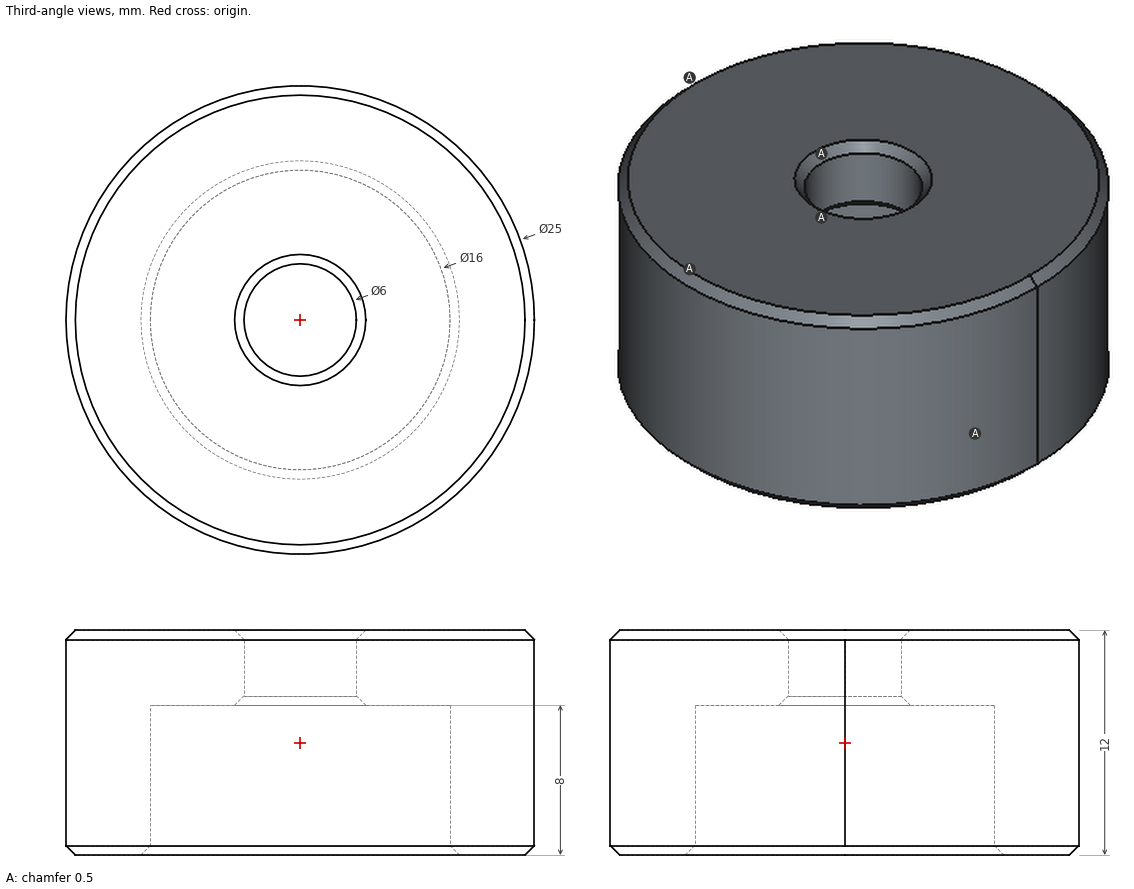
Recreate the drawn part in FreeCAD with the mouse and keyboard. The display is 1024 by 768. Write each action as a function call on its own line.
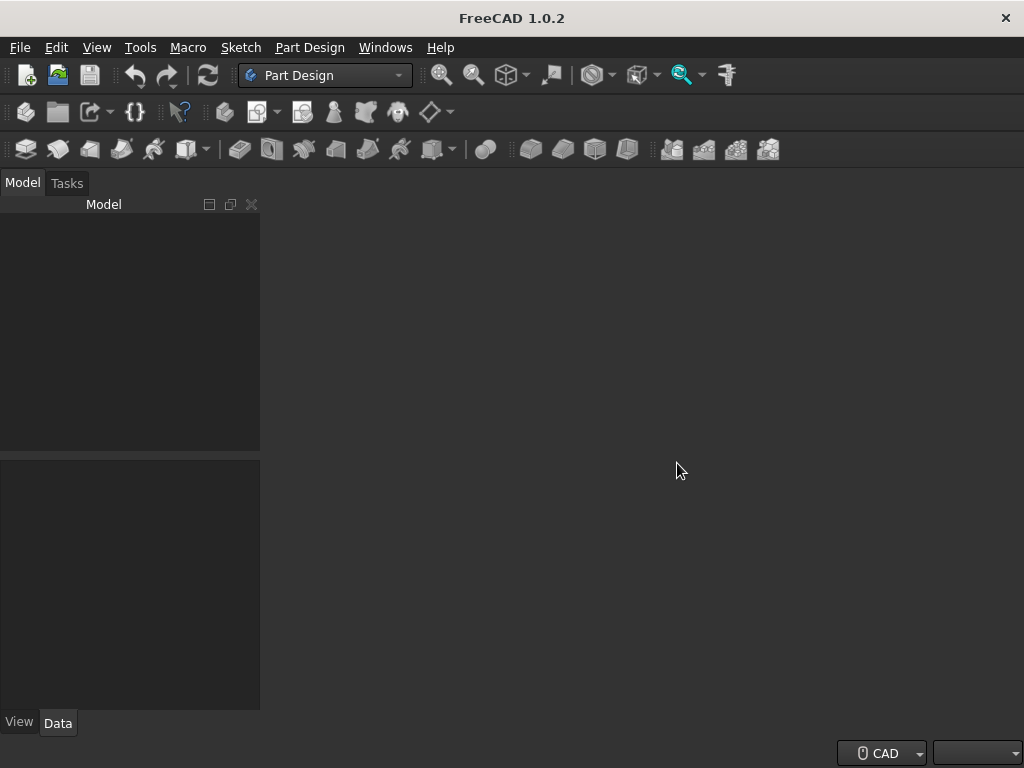
key(ctrl+n)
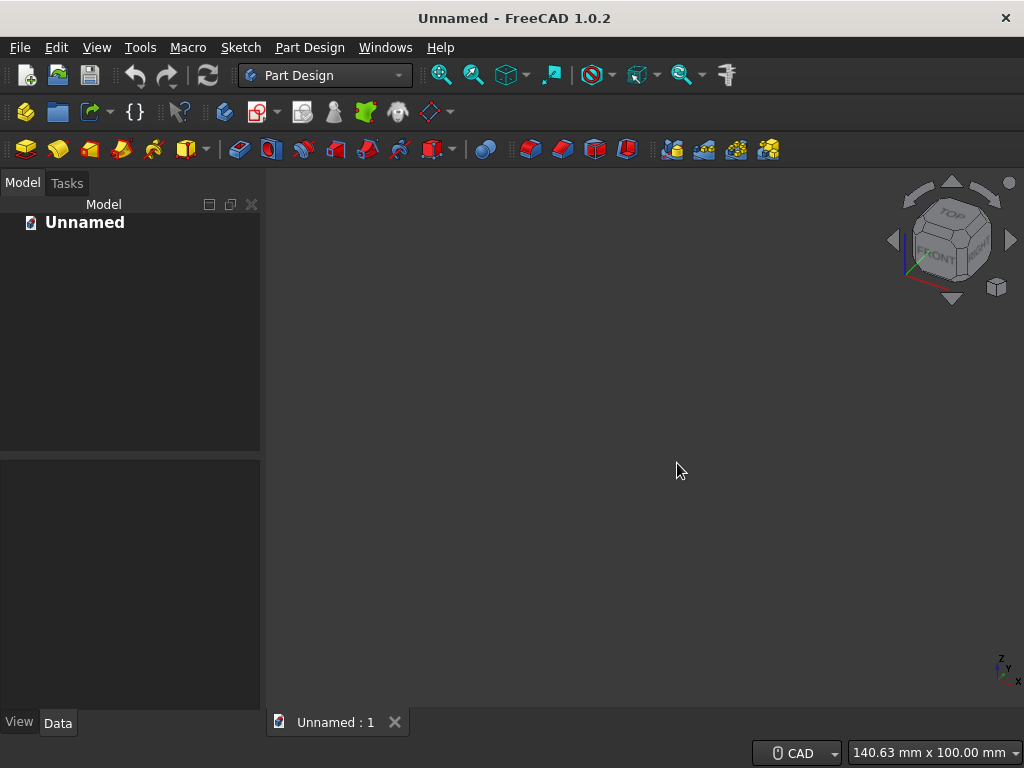
click(258, 112)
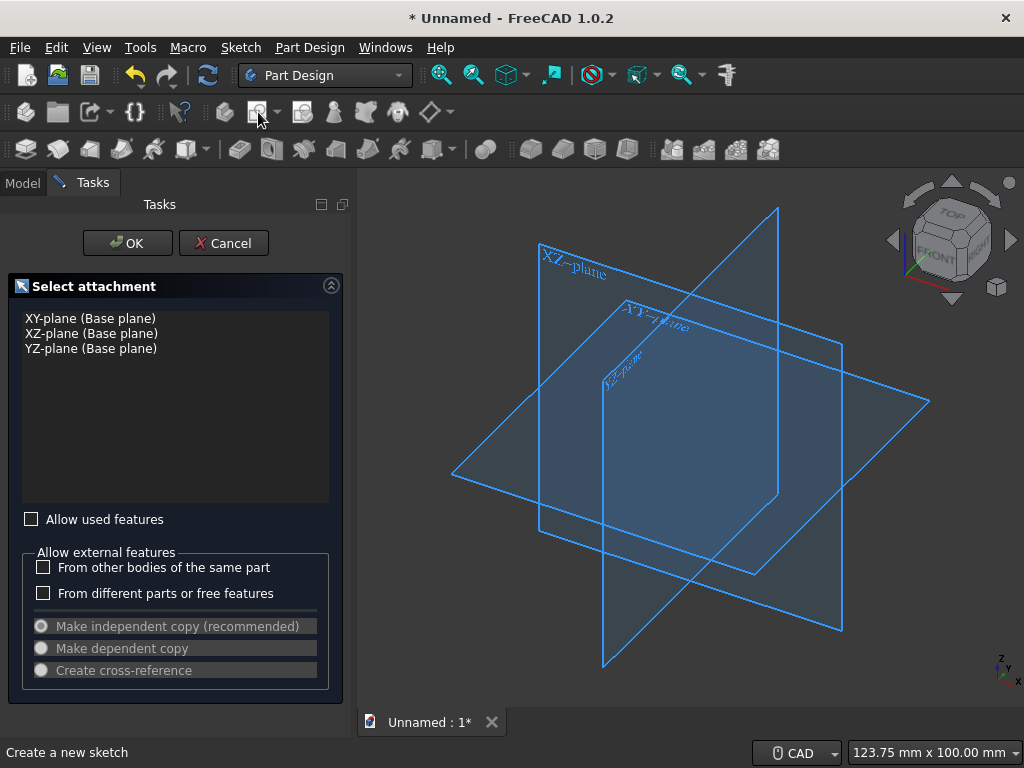
click(82, 318)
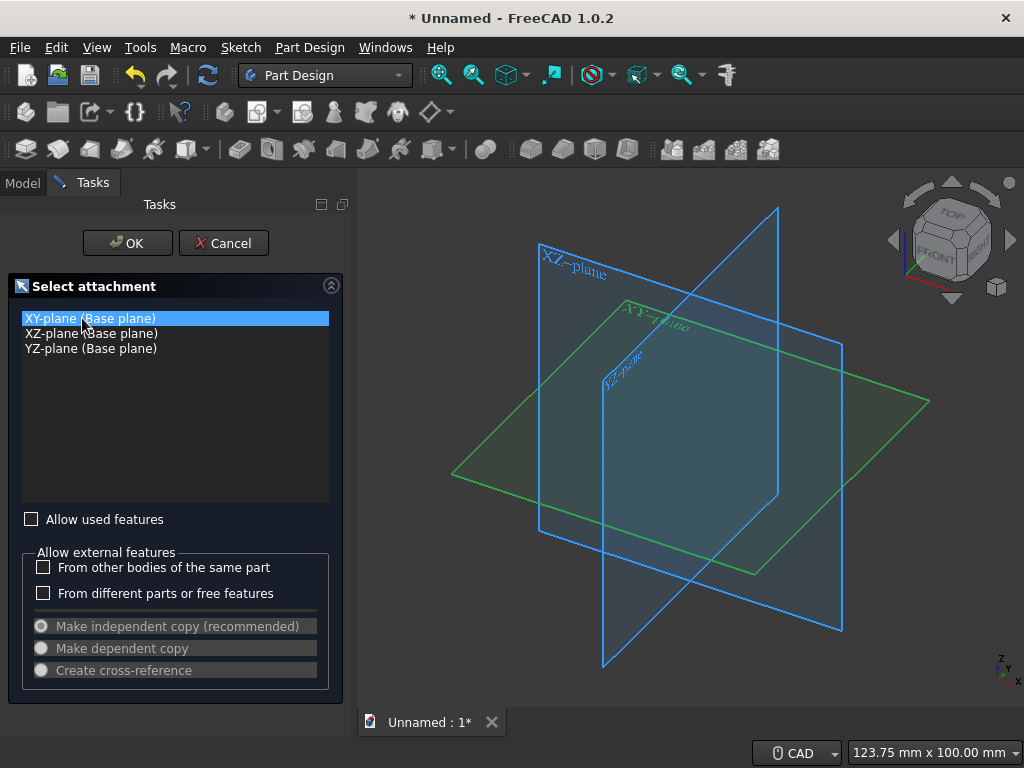
click(128, 243)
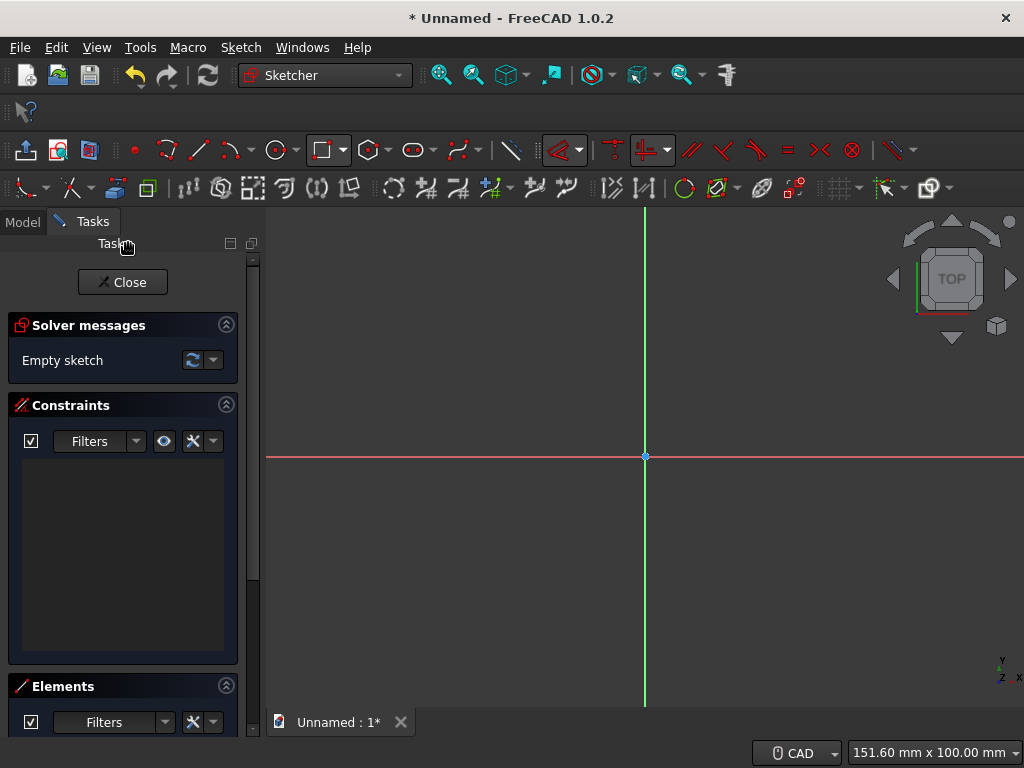
scroll(685, 457, up, 5)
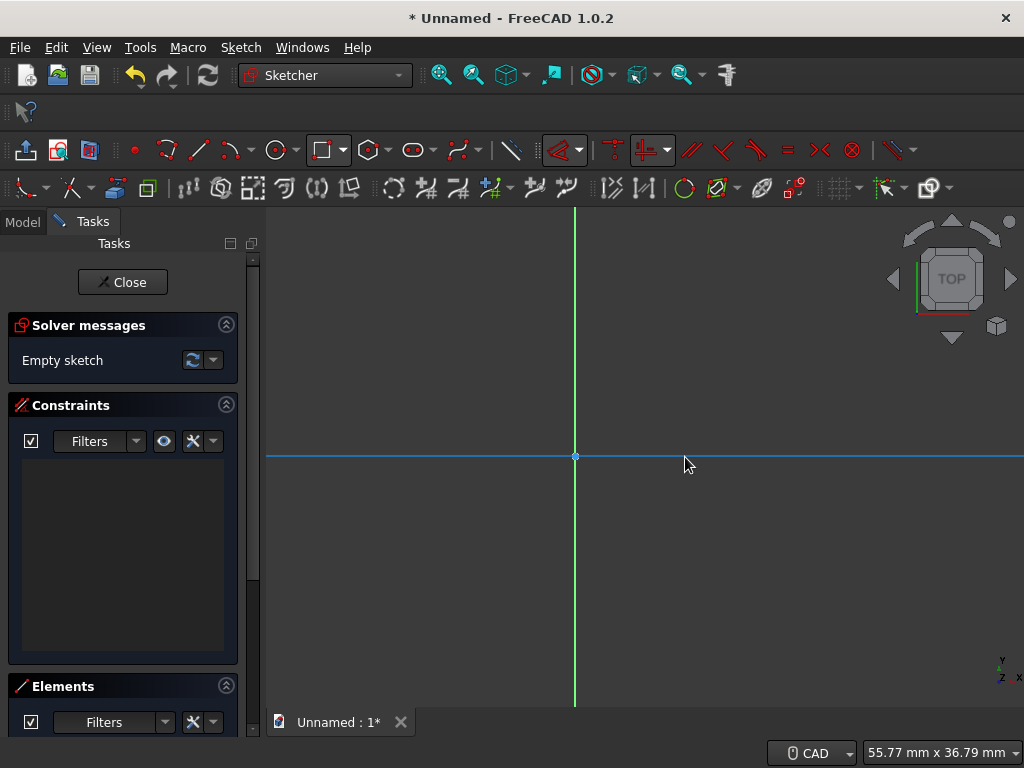
key(g)
key(c)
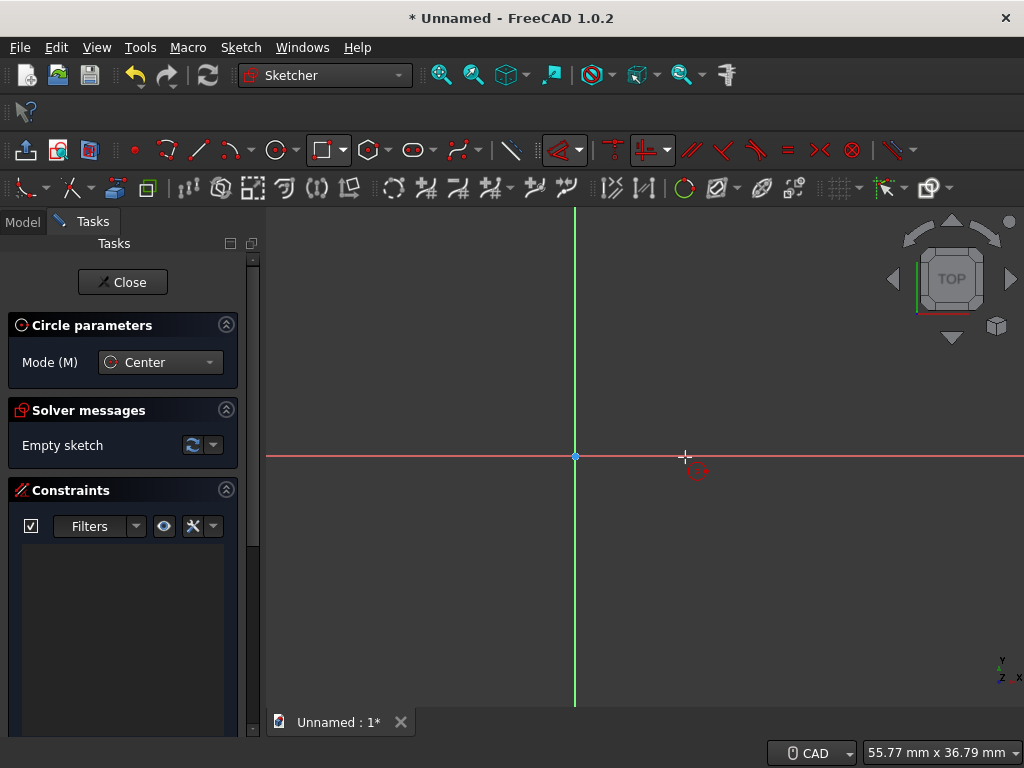
click(575, 456)
move(695, 336)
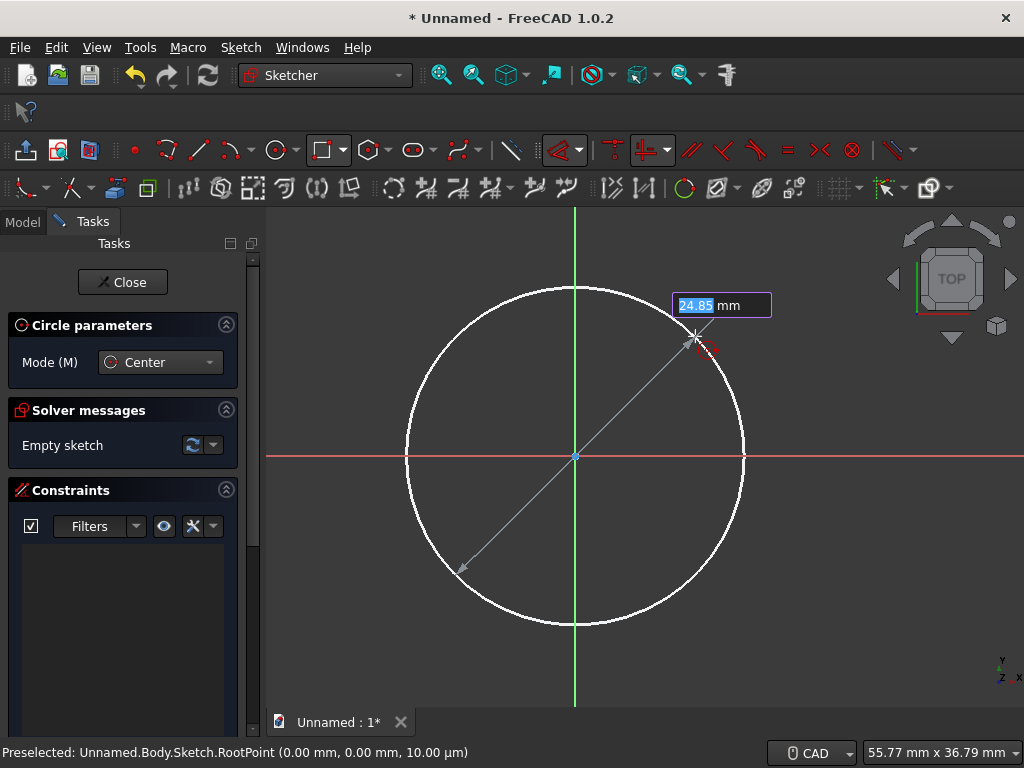
text(25)
key(Return)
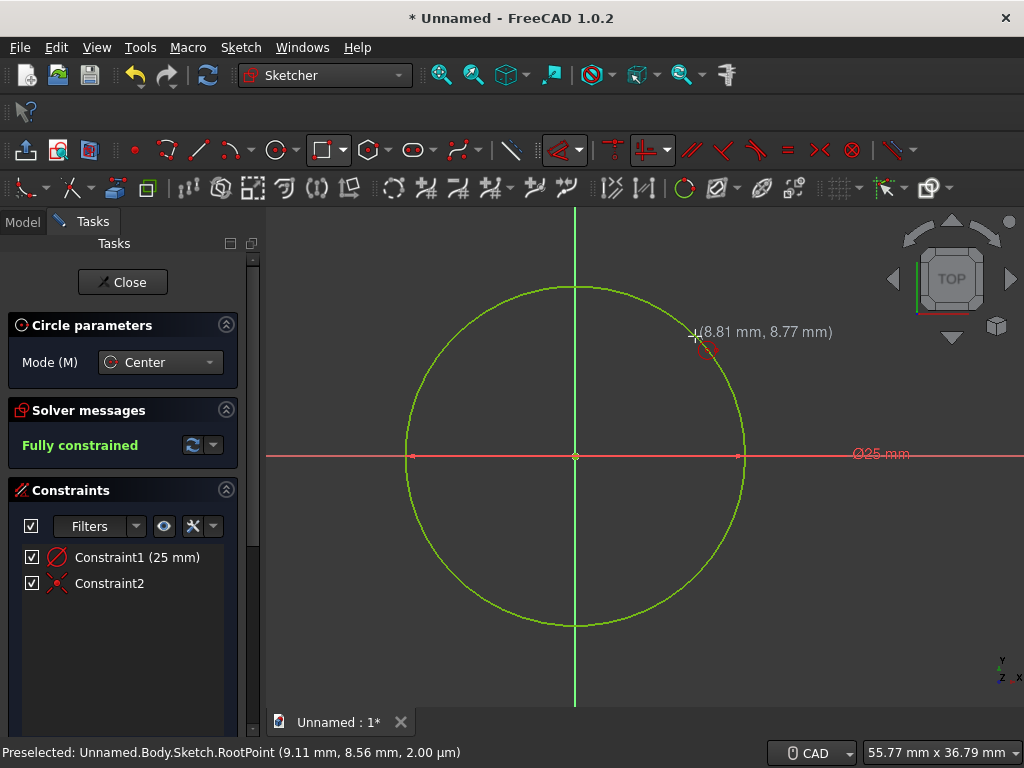
click(575, 456)
move(604, 427)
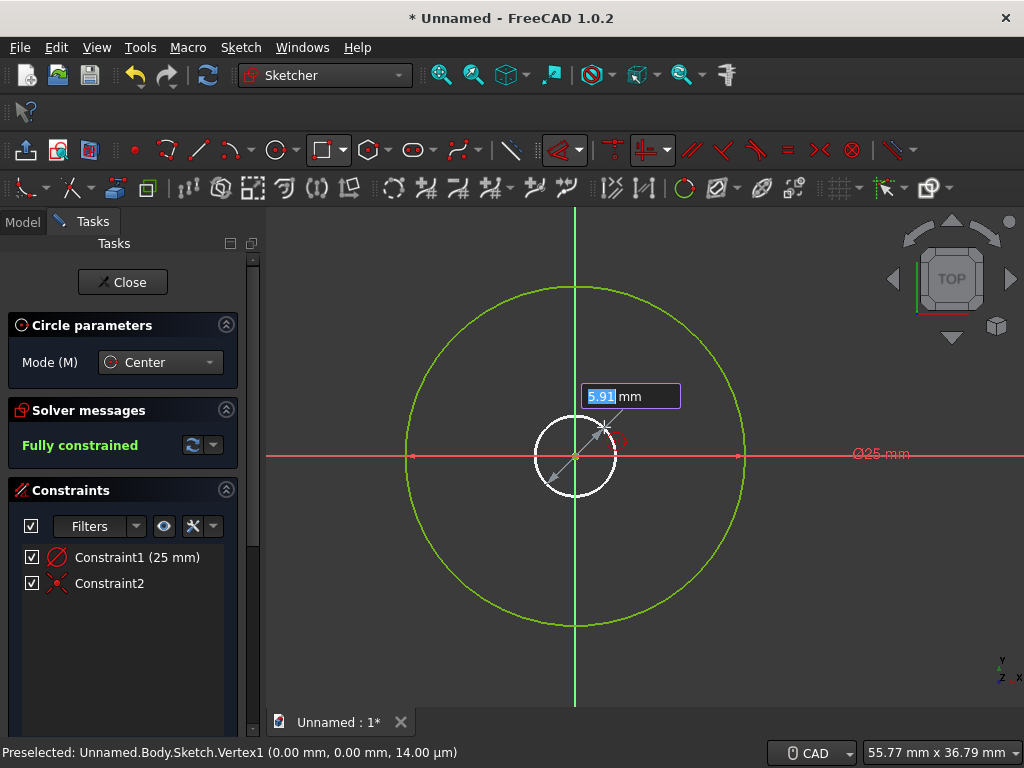
text(6)
key(Return)
key(Escape)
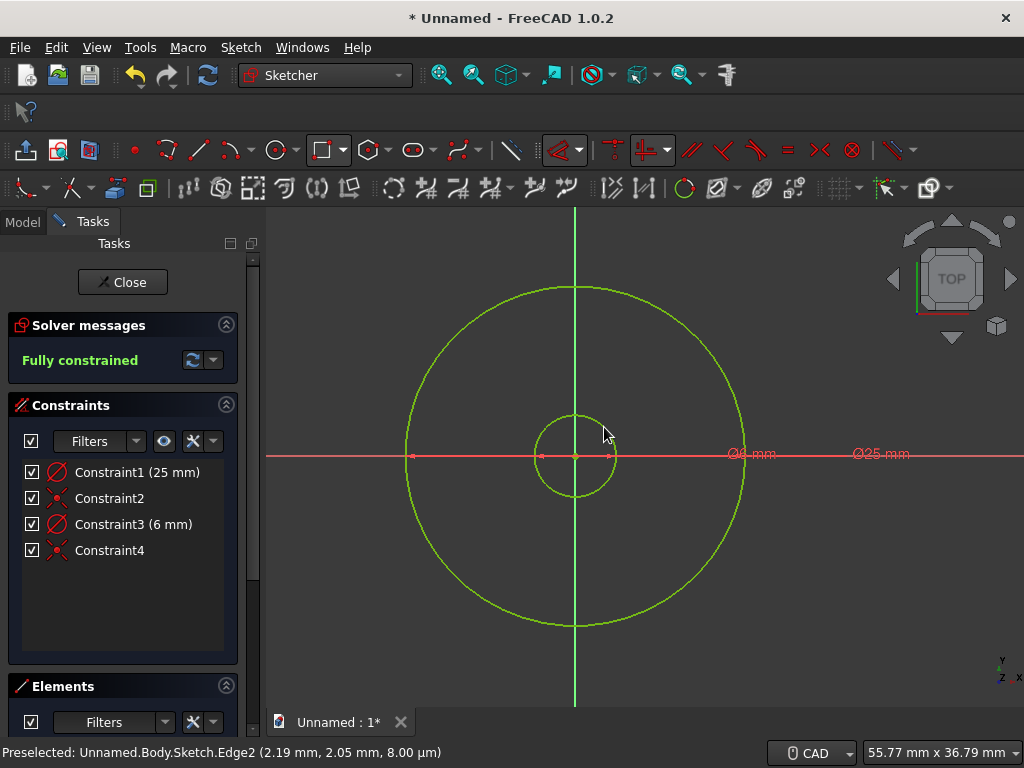
click(123, 282)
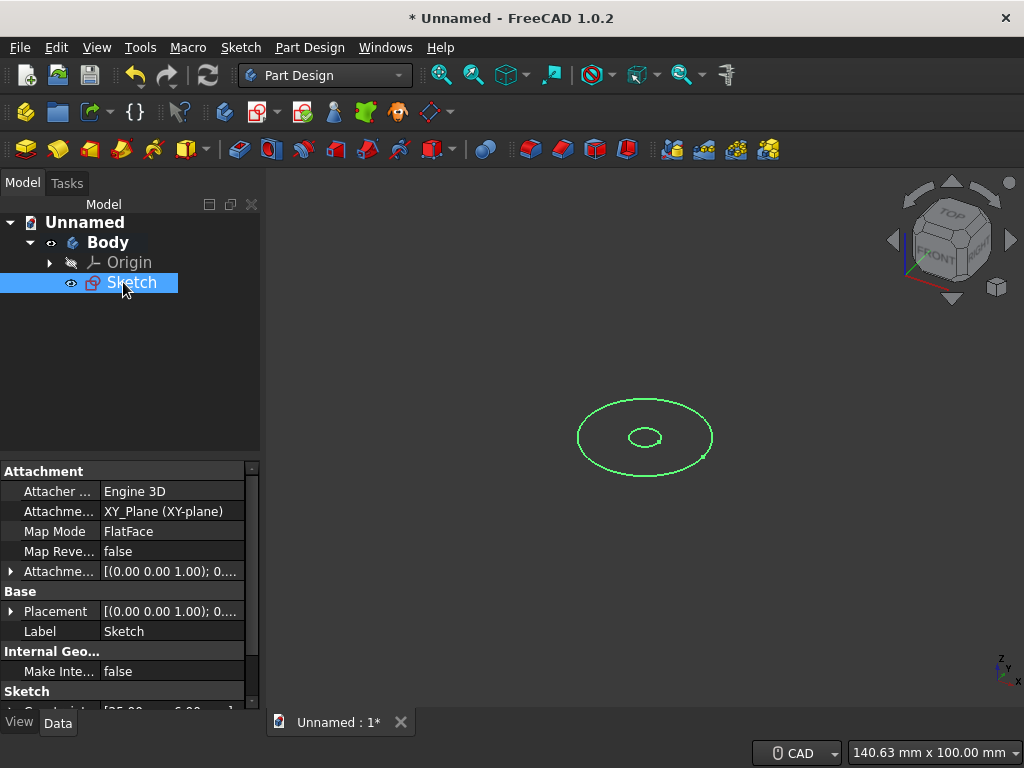
click(26, 150)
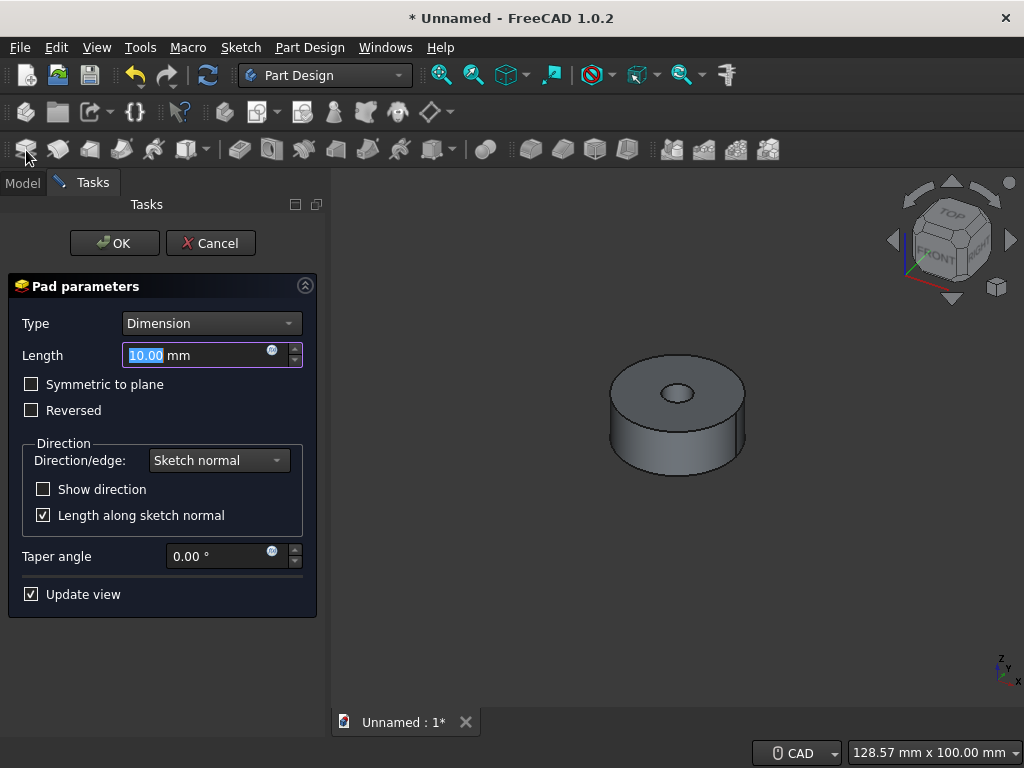
text(12)
key(Tab)